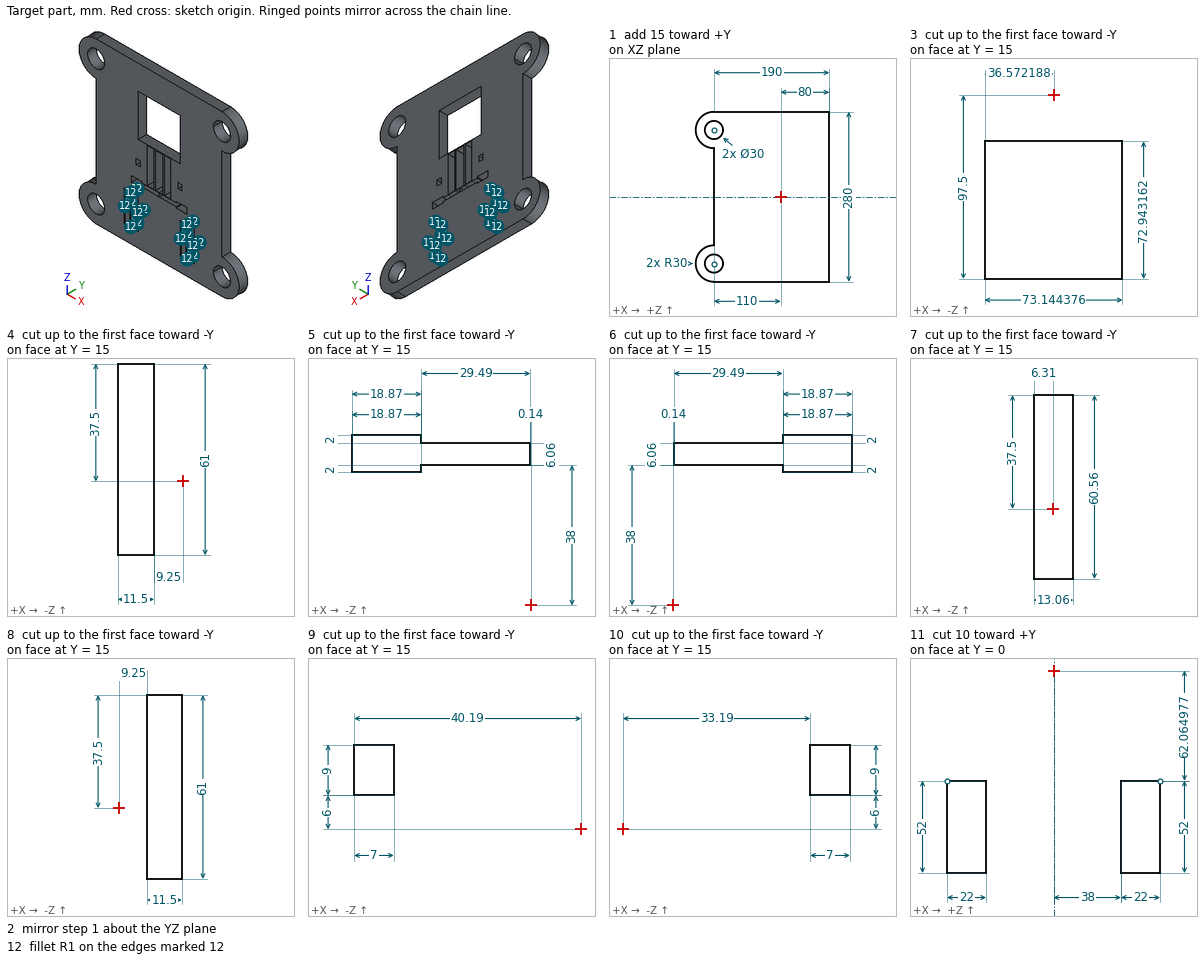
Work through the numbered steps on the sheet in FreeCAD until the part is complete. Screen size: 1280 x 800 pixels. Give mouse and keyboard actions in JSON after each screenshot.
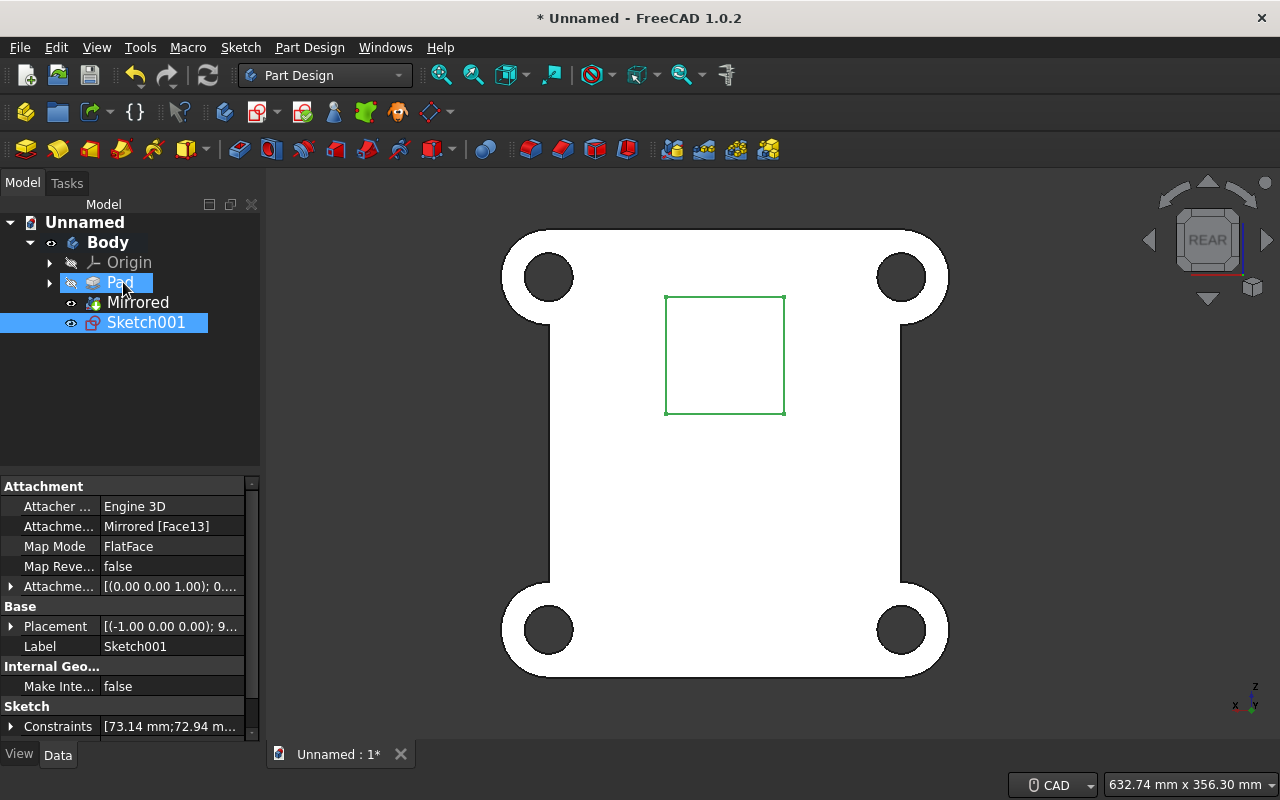
{"action": "left_click", "coordinate": [240, 150]}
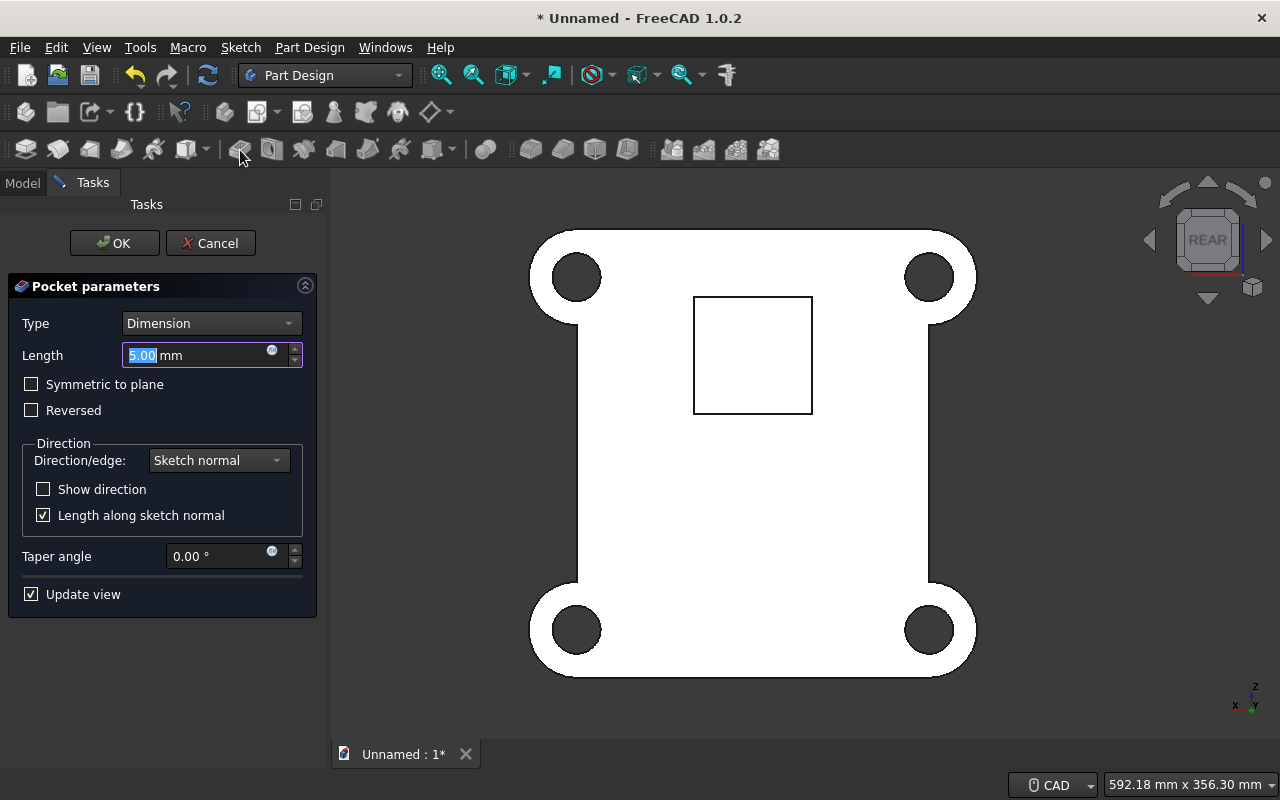
{"action": "left_click", "coordinate": [212, 324]}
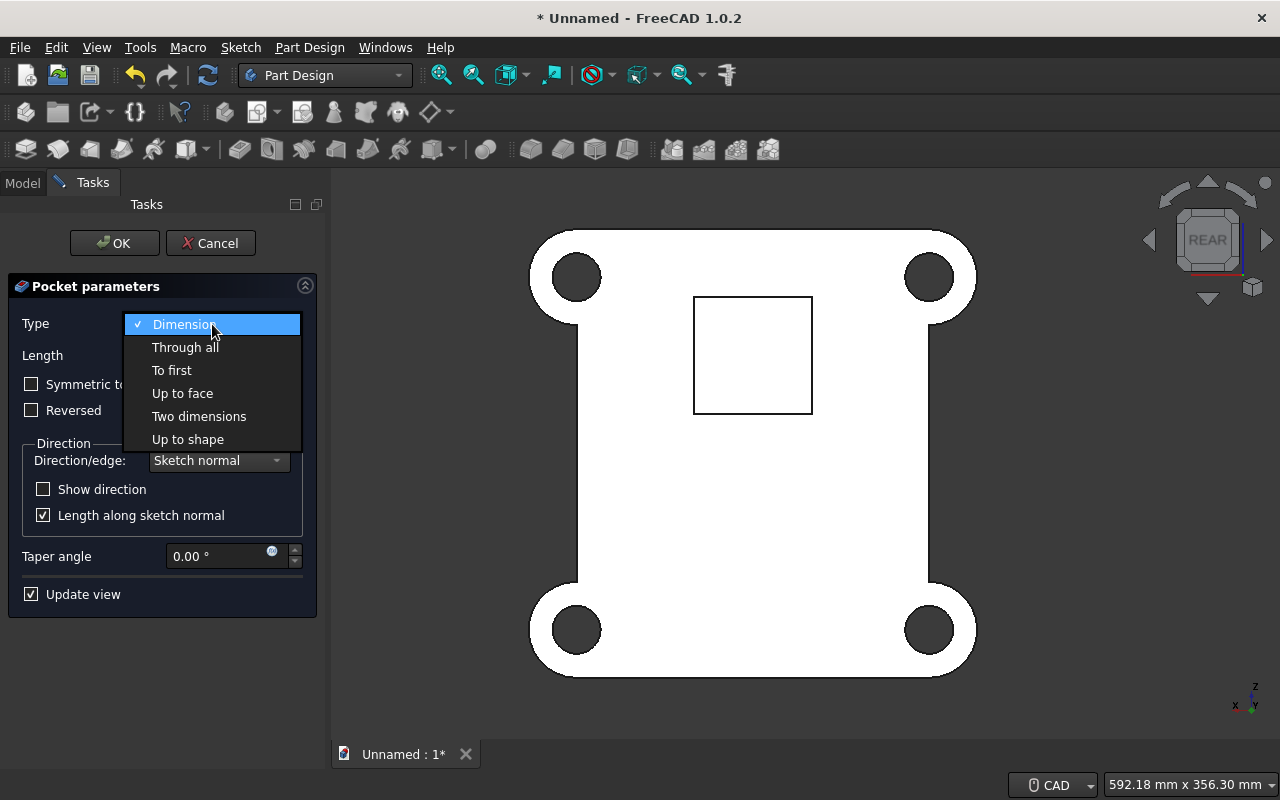
{"action": "left_click", "coordinate": [212, 370]}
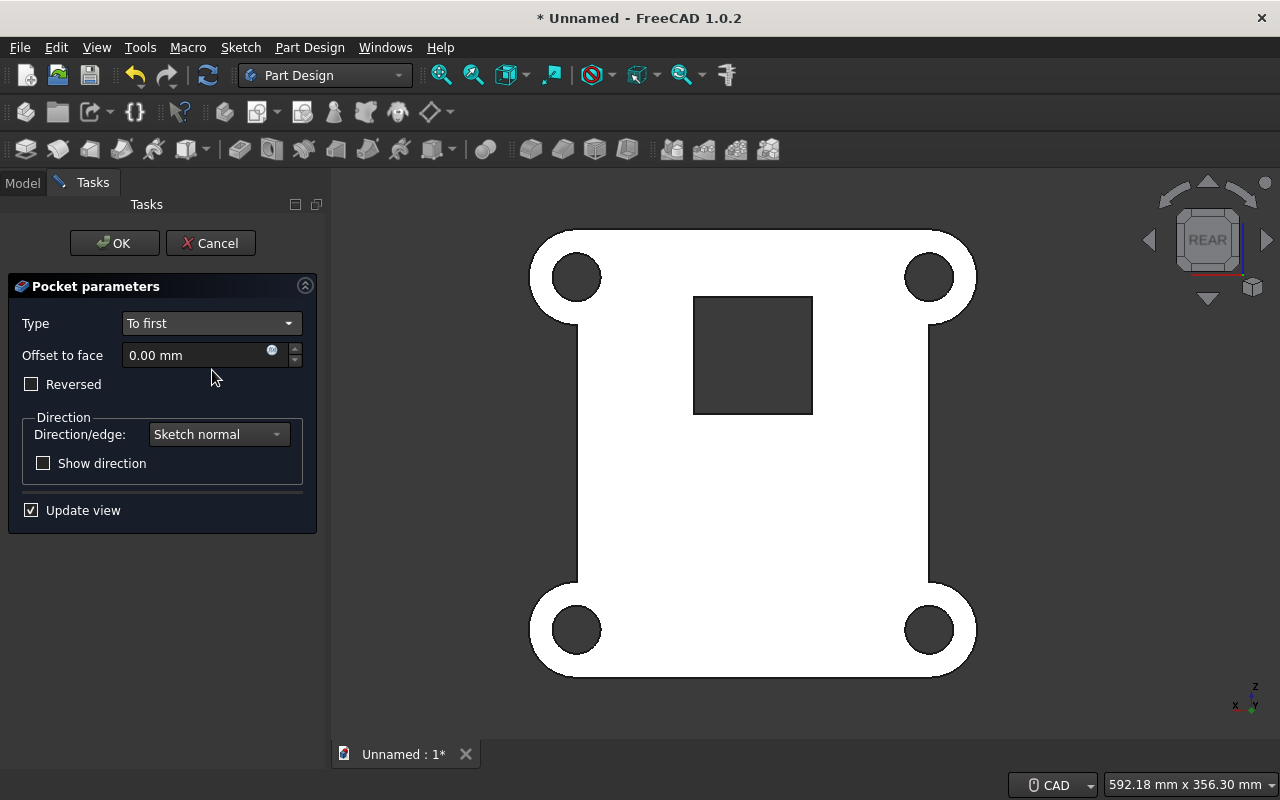
{"action": "left_click", "coordinate": [115, 243]}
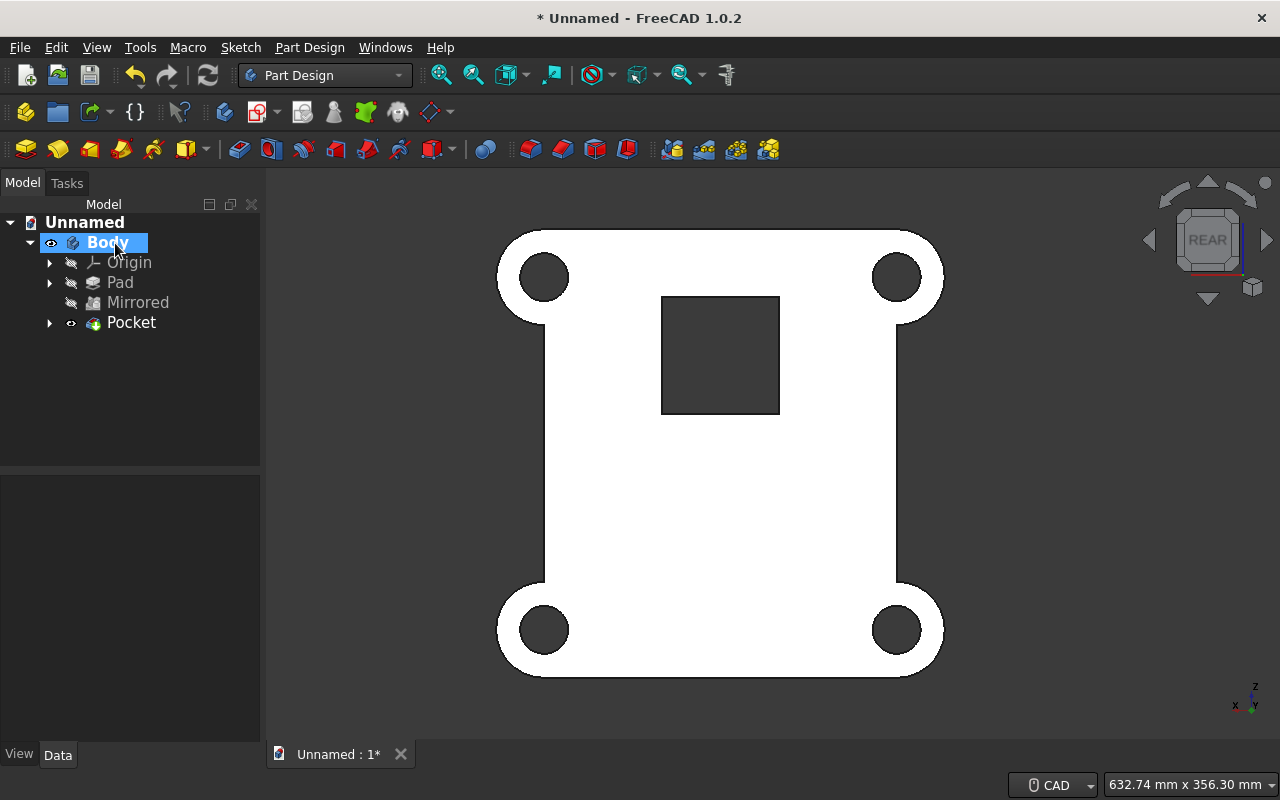
{"action": "left_click", "coordinate": [656, 517]}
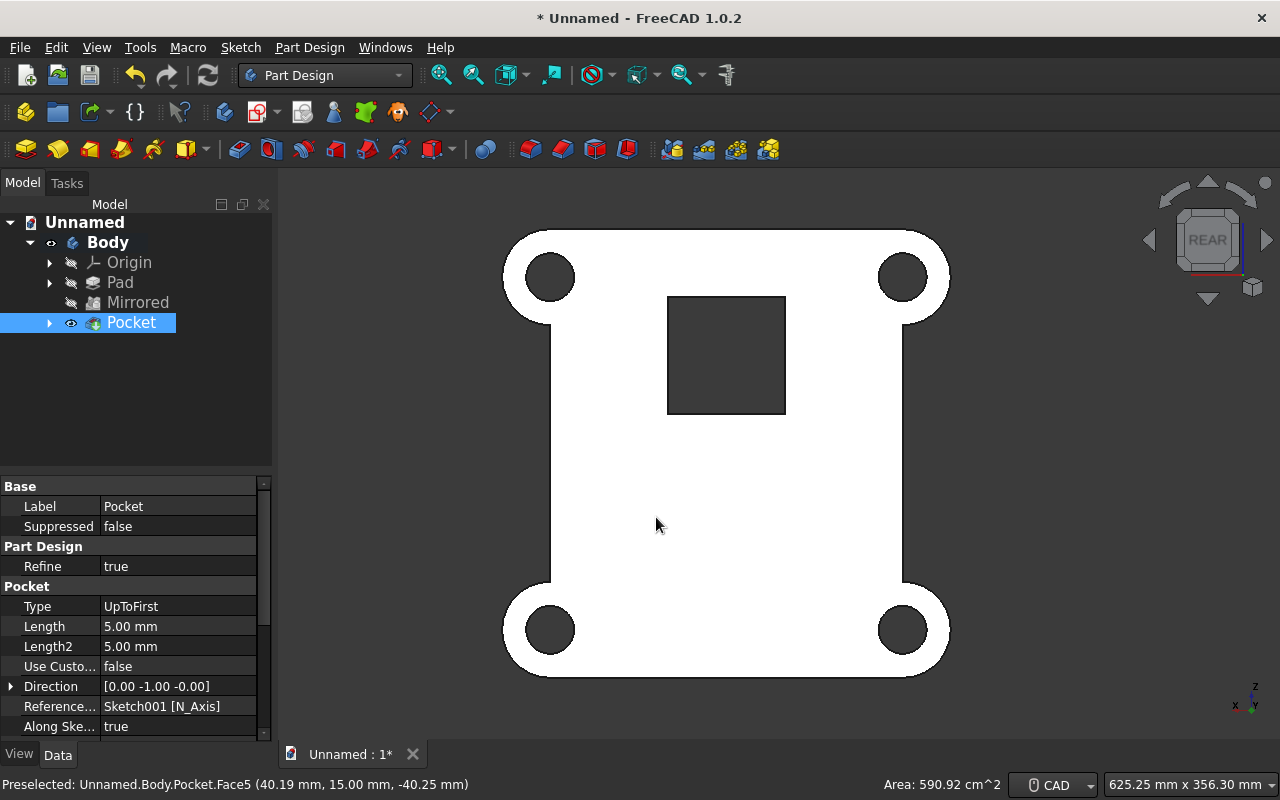
{"action": "left_click", "coordinate": [258, 112]}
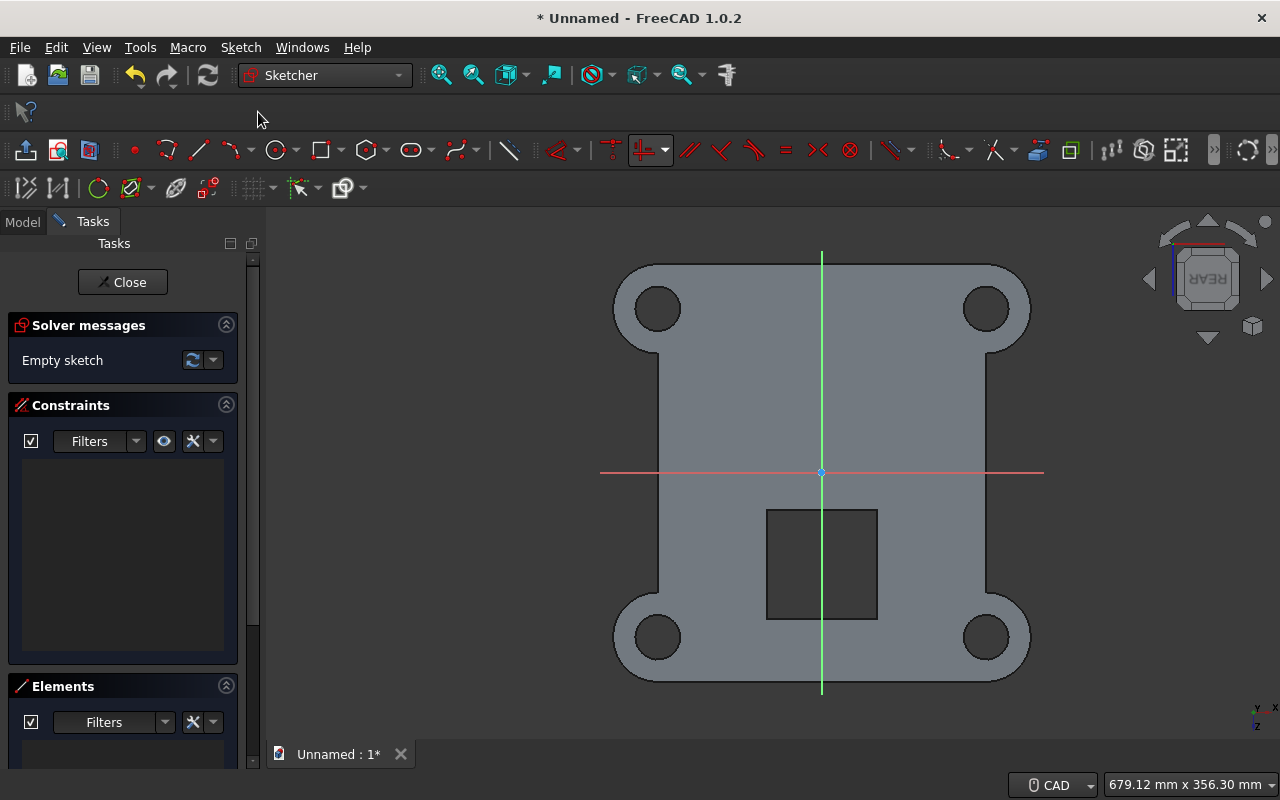
{"action": "scroll", "coordinate": [840, 459], "scroll_direction": "up", "scroll_amount": 7}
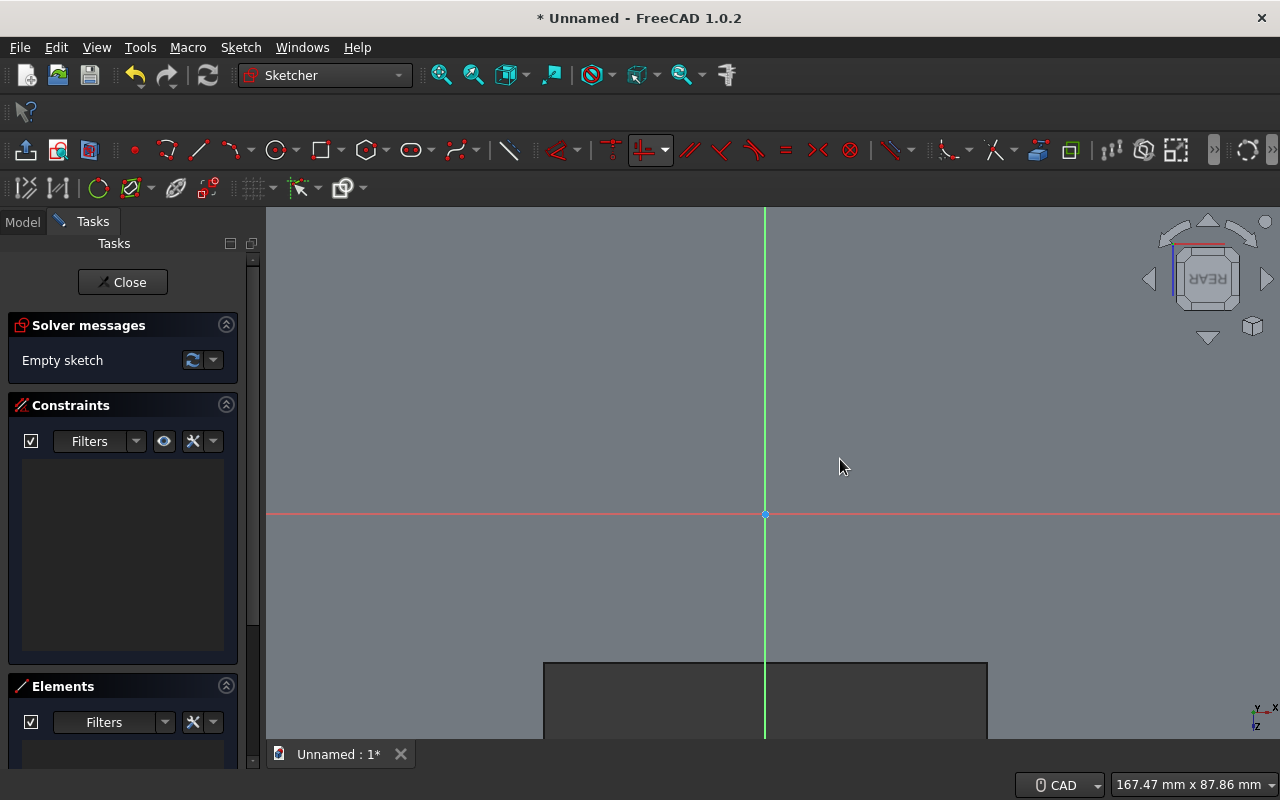
{"action": "key", "text": "g r"}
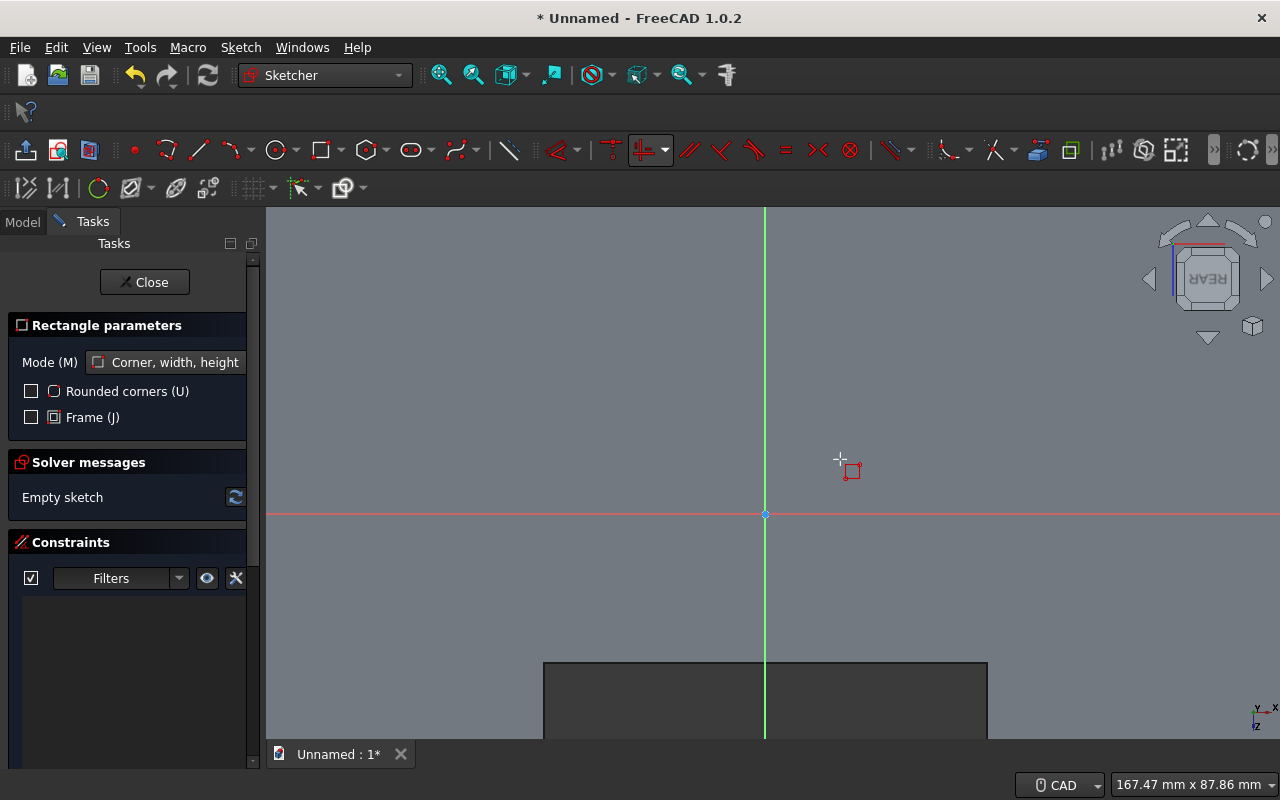
{"action": "left_click", "coordinate": [640, 287]}
{"action": "mouse_move", "coordinate": [709, 657]}